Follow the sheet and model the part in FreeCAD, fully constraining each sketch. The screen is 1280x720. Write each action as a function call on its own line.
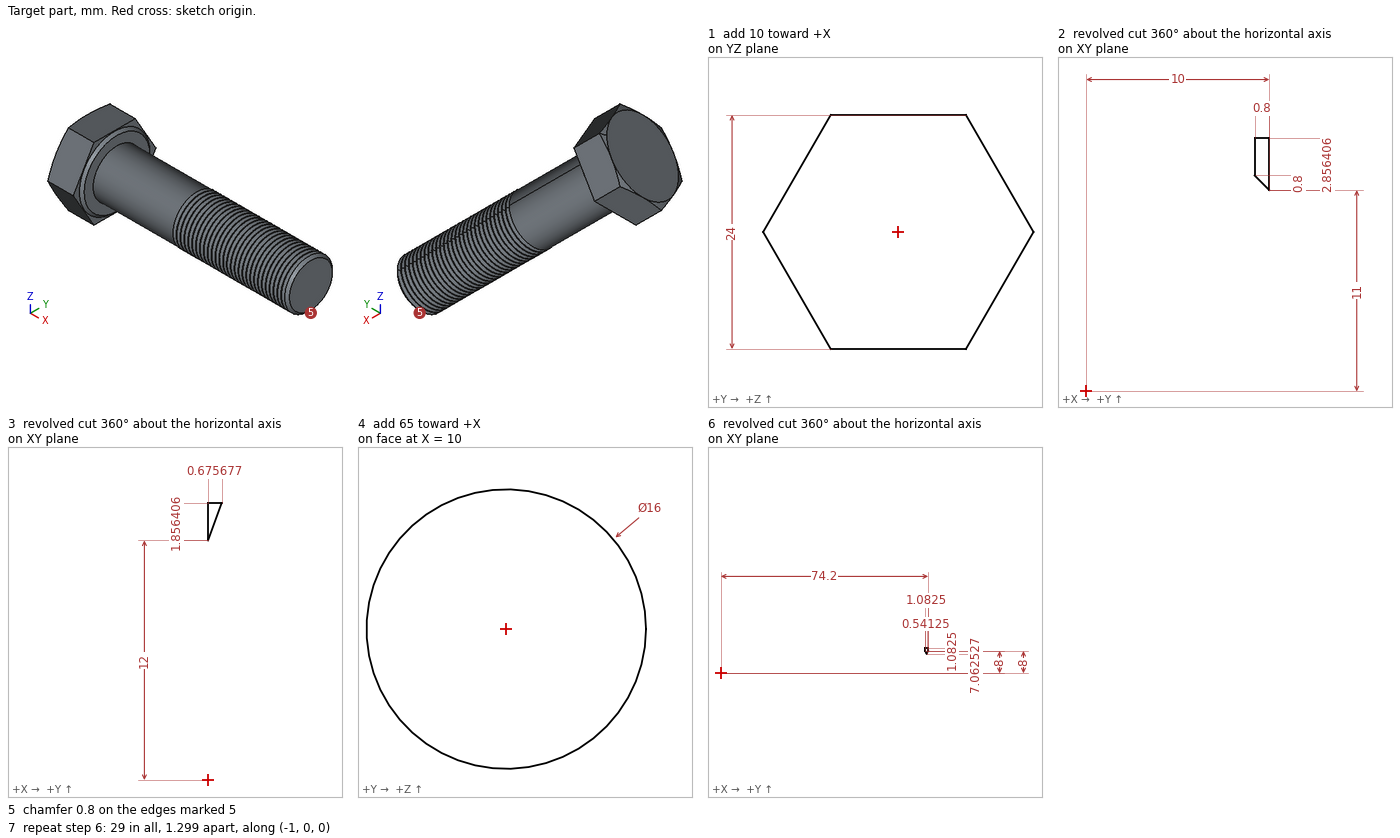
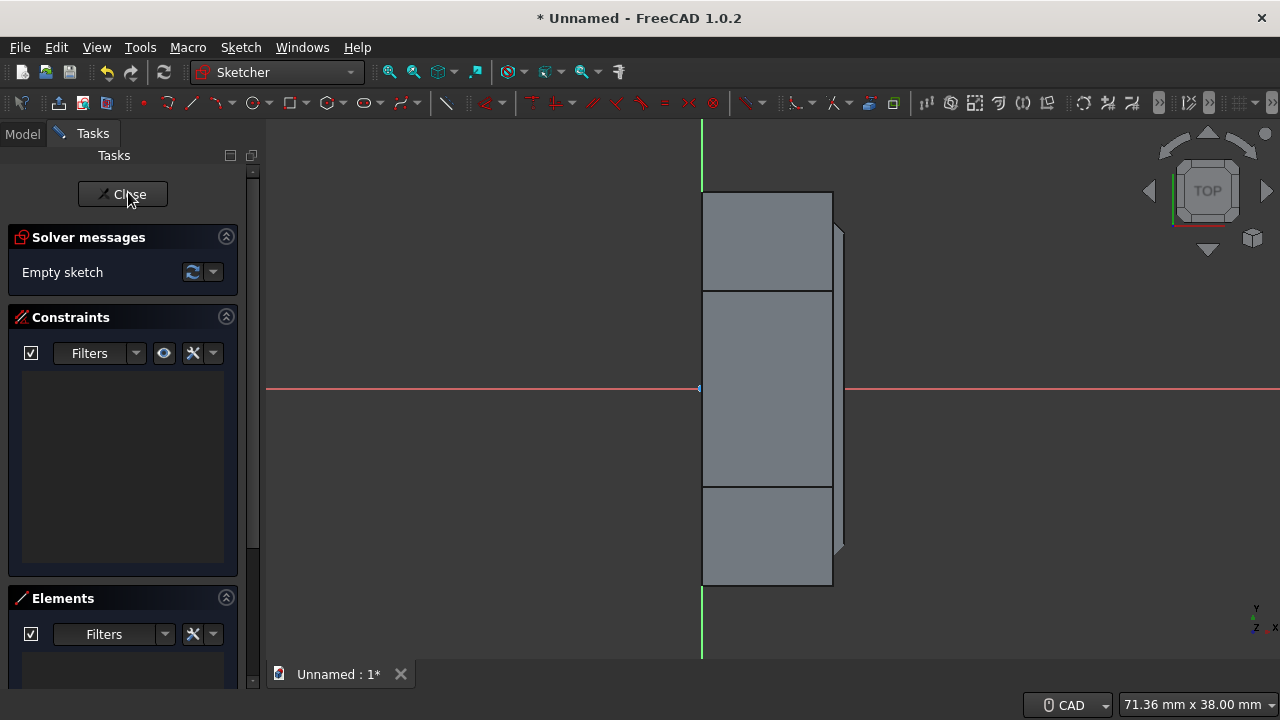
click(108, 104)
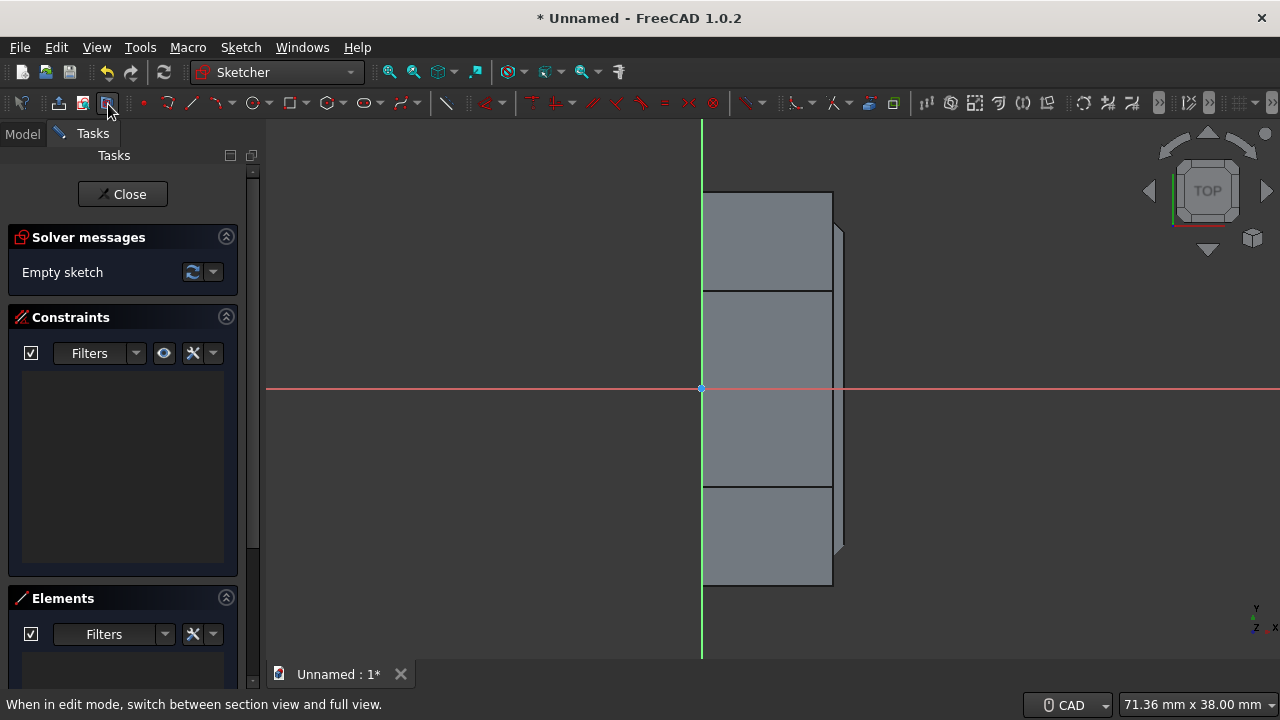
scroll(707, 191, up, 13)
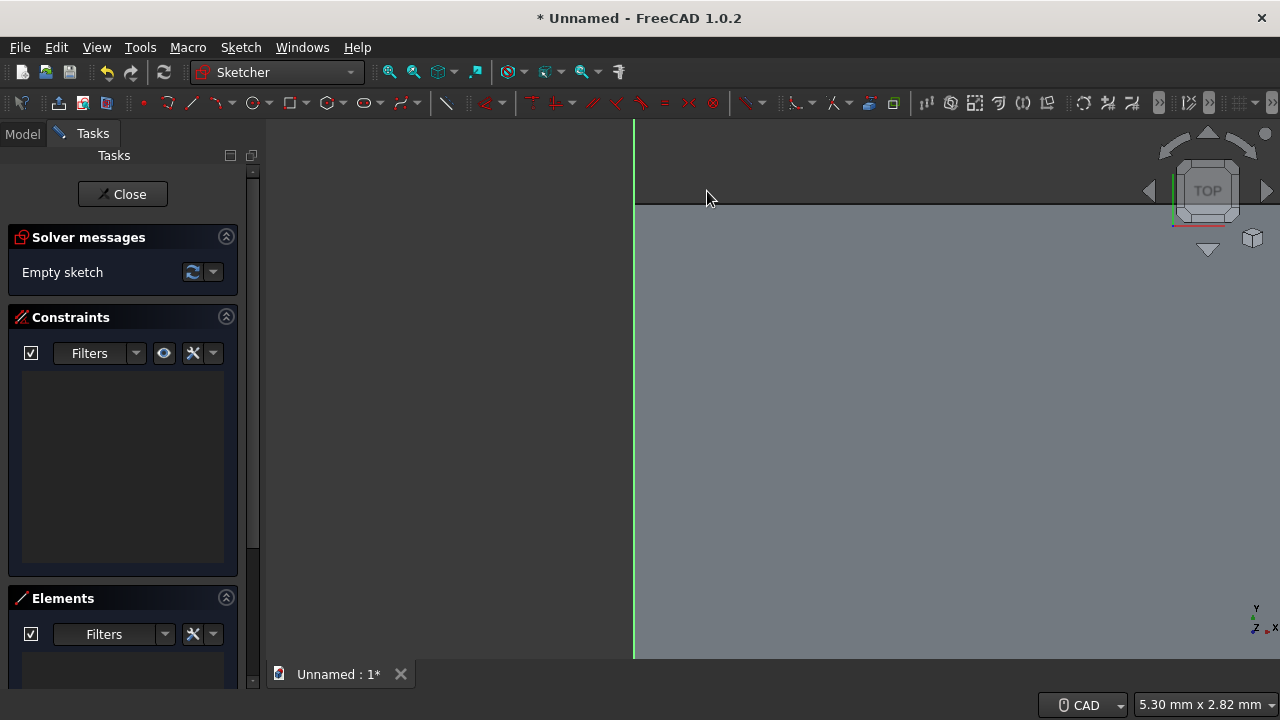
click(168, 104)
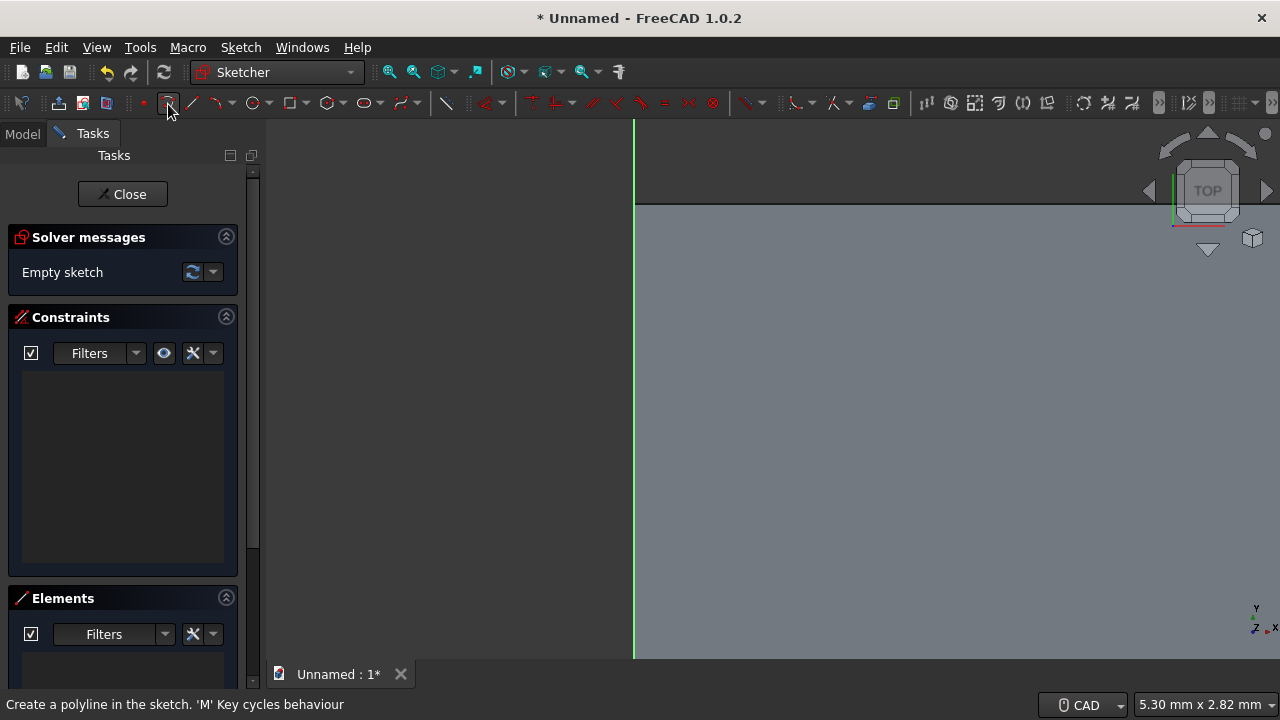
click(634, 559)
click(763, 204)
click(643, 204)
click(634, 560)
key(Escape)
key(Escape)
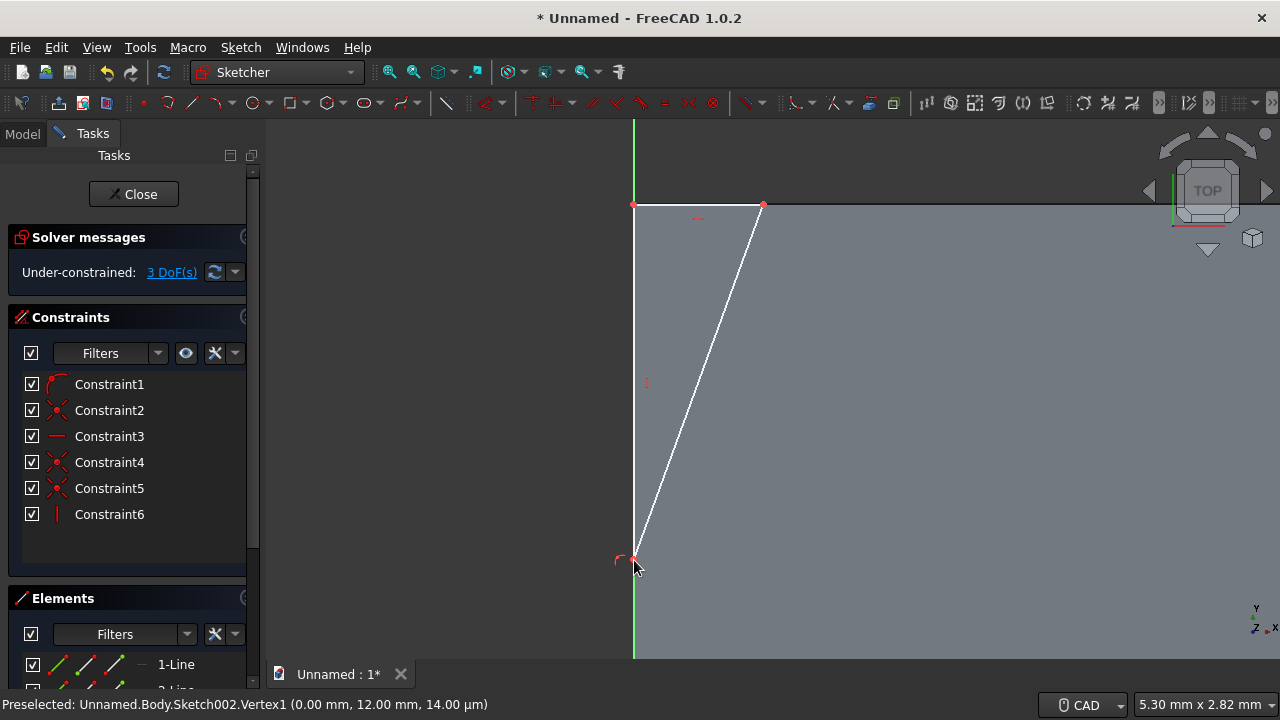
click(486, 104)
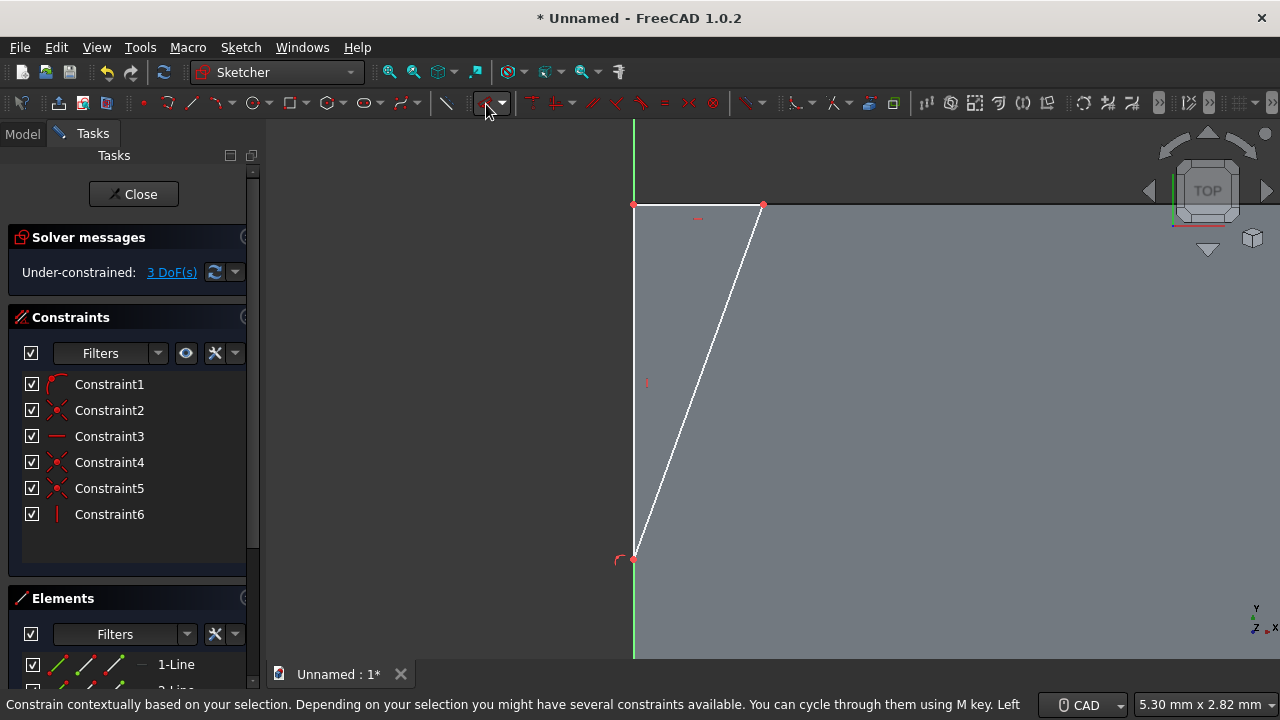
click(634, 560)
click(600, 595)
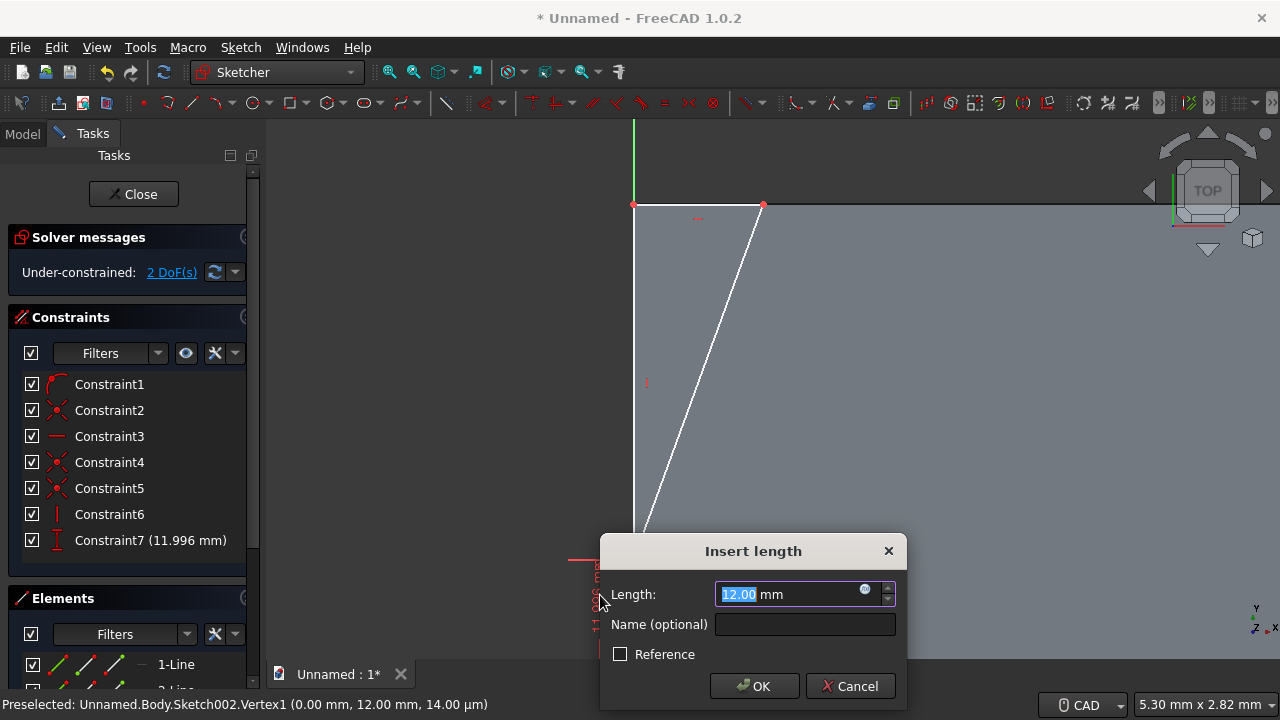
text(12)
key(Return)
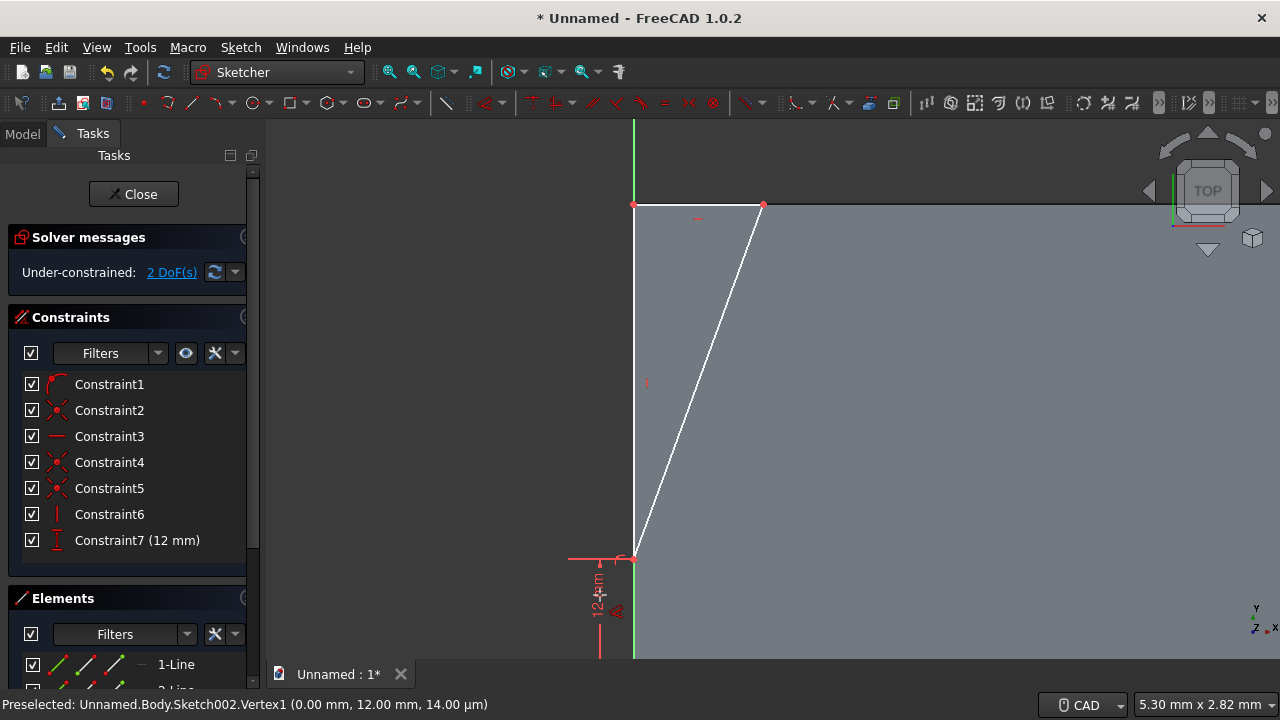
click(724, 205)
click(698, 171)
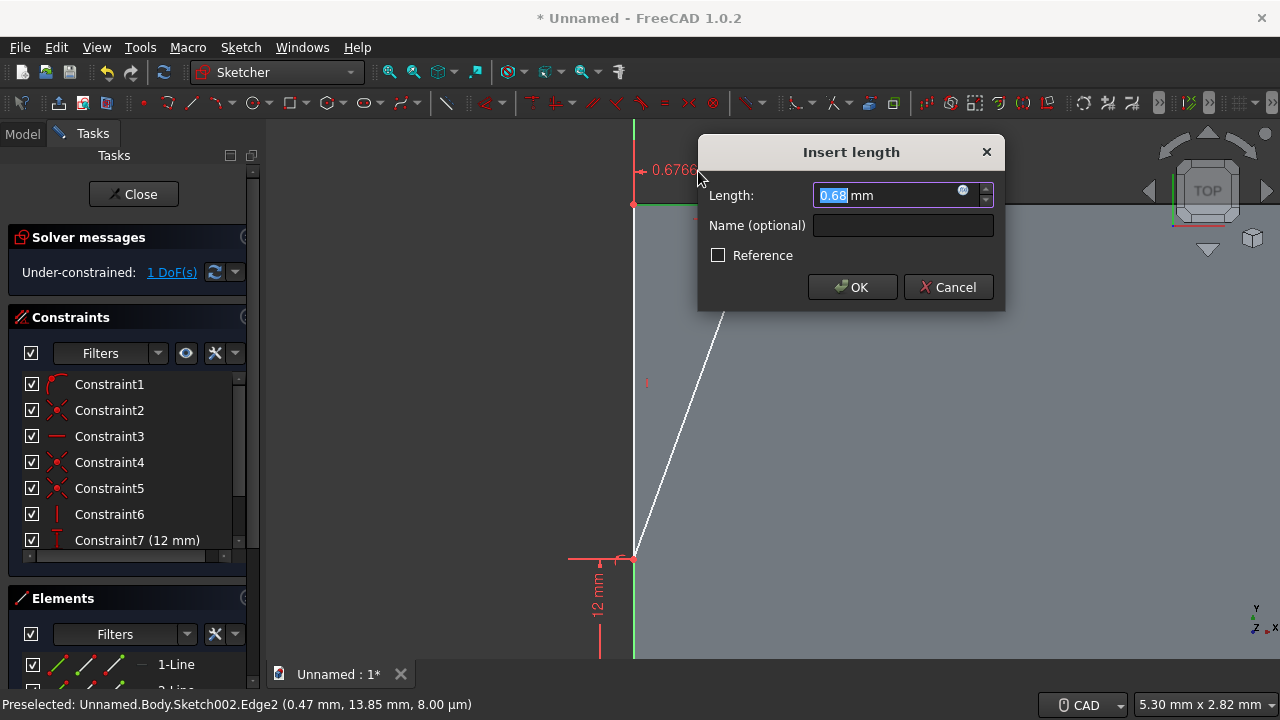
text(0.675677)
key(Return)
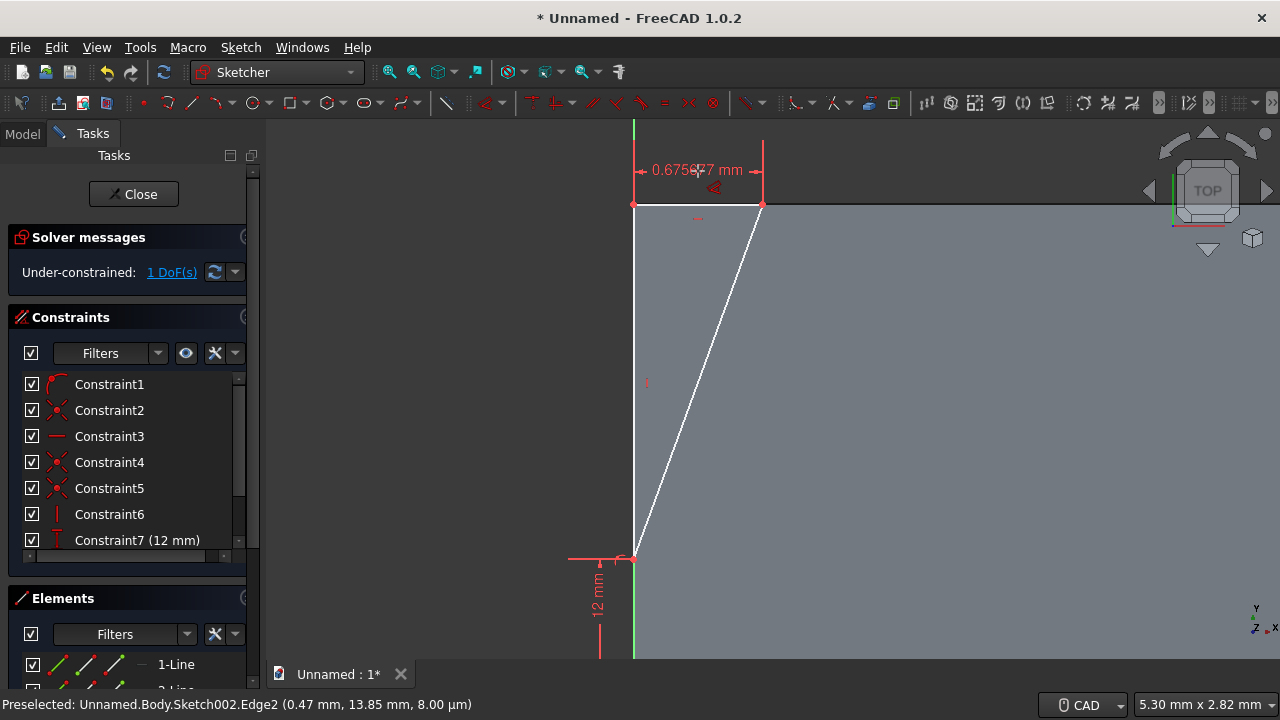
click(634, 311)
click(600, 382)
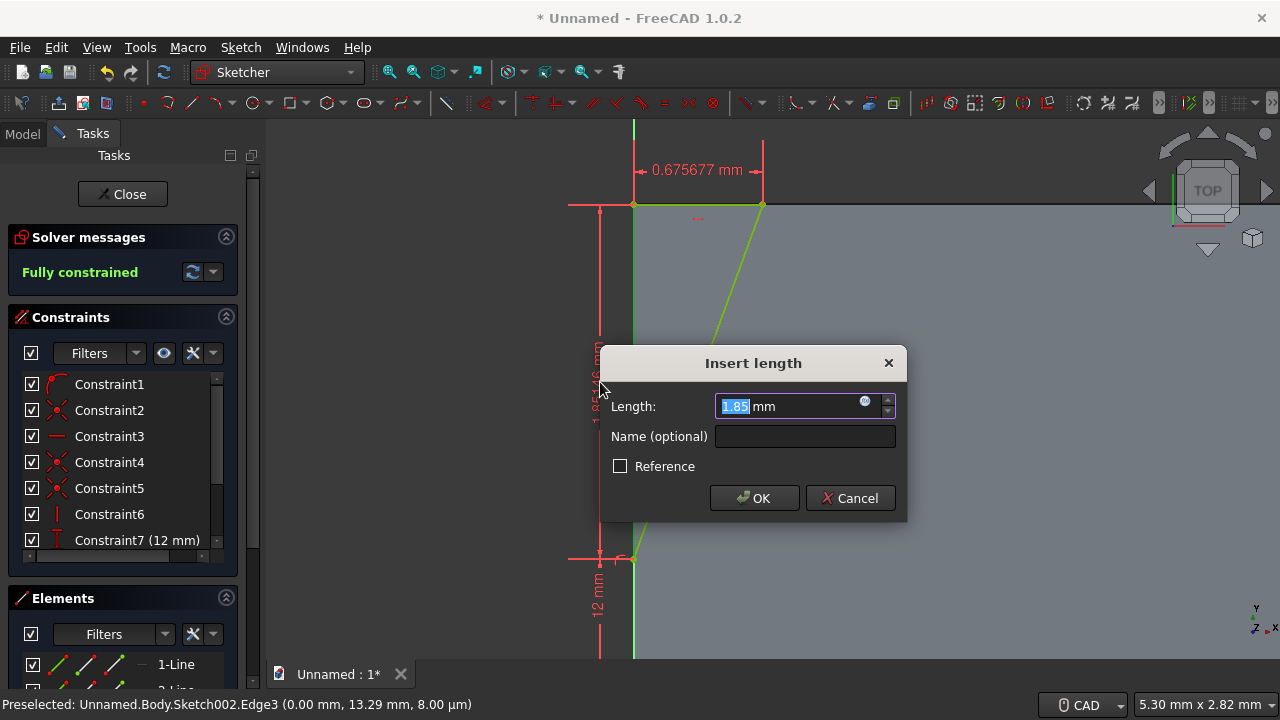
text(1.856406)
key(Return)
key(Escape)